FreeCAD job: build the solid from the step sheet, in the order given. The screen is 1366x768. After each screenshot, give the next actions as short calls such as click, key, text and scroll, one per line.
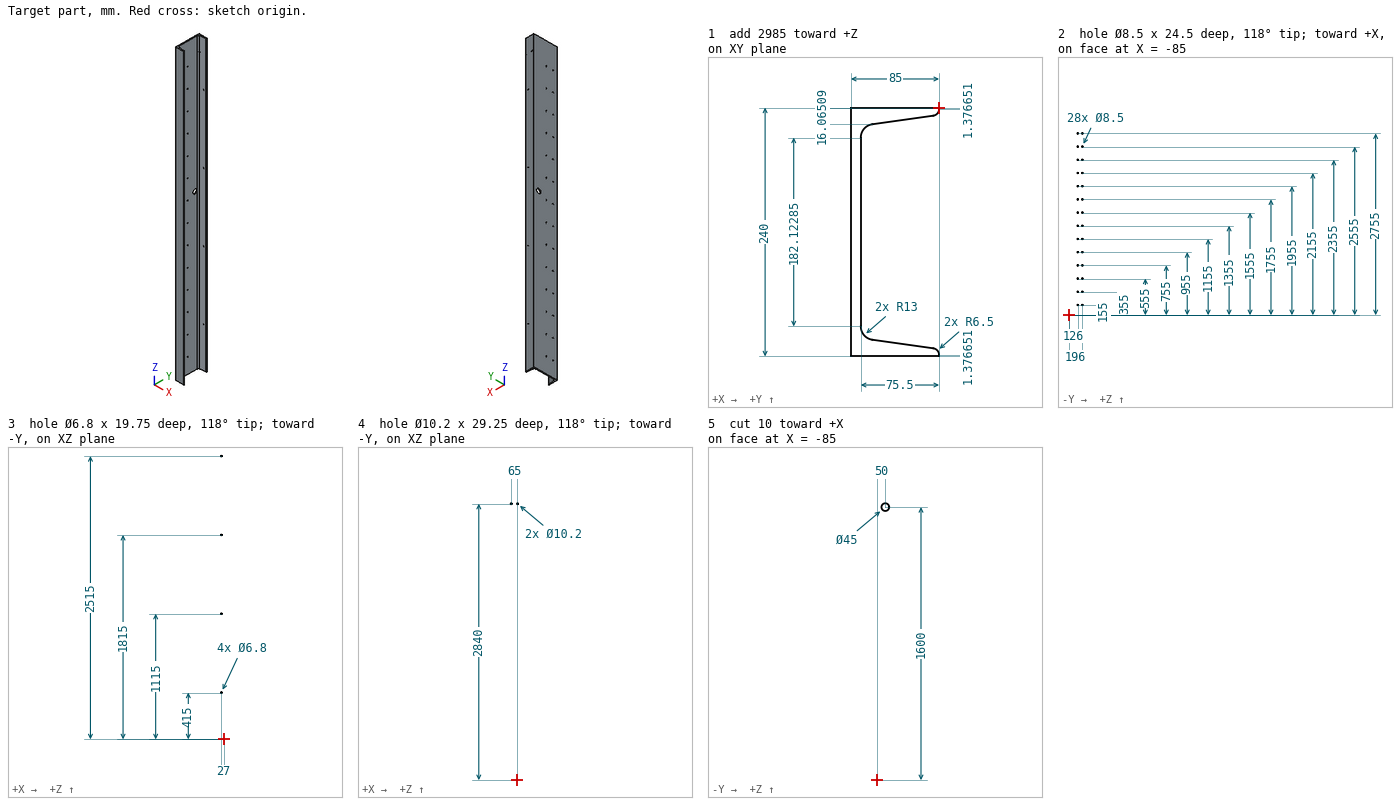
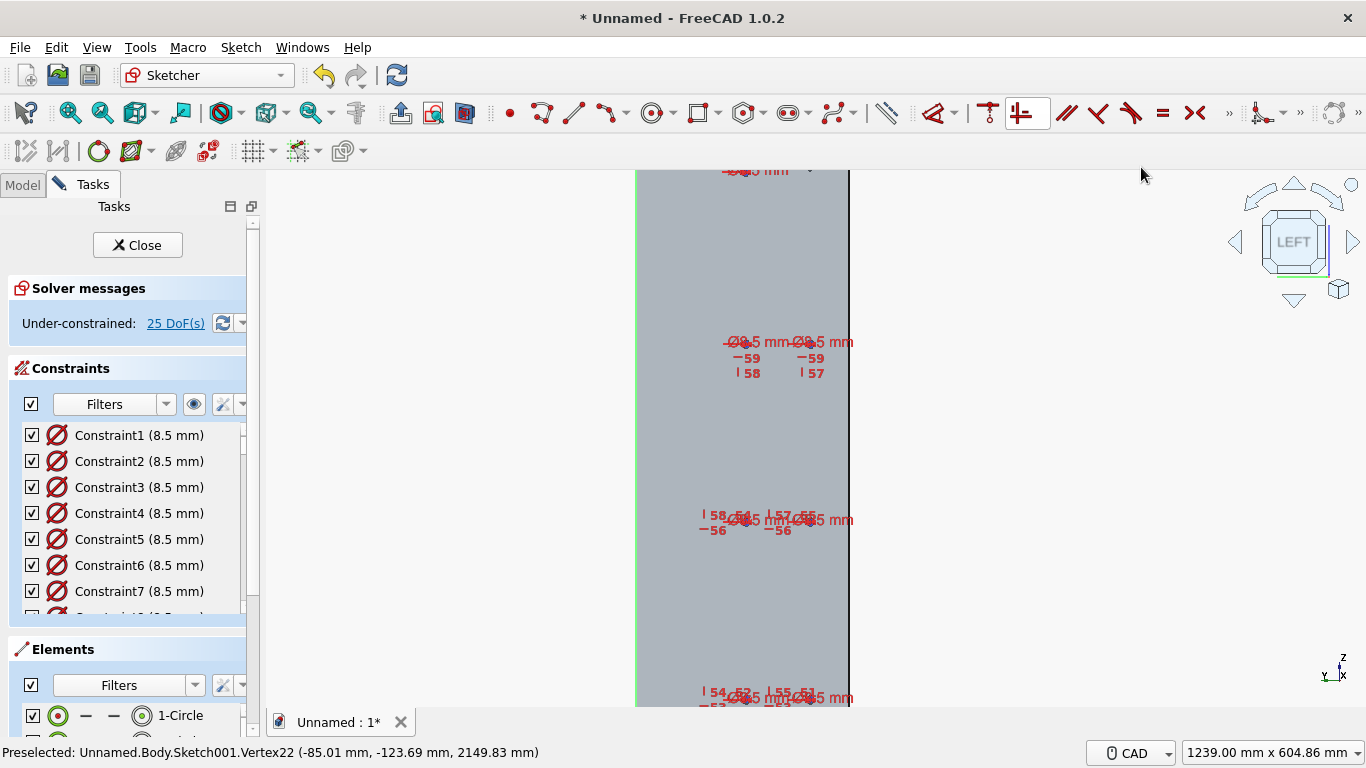
scroll(751, 346, down, 10)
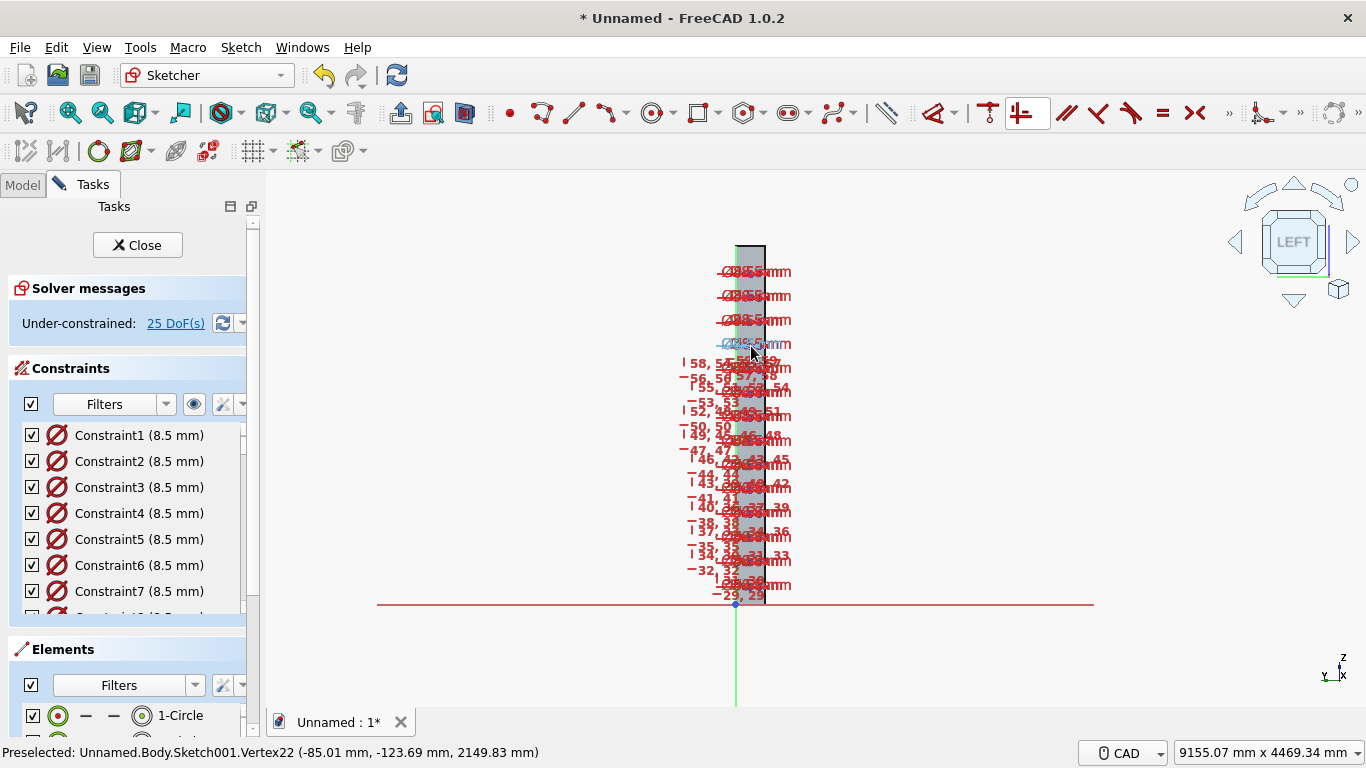
scroll(751, 346, up, 2)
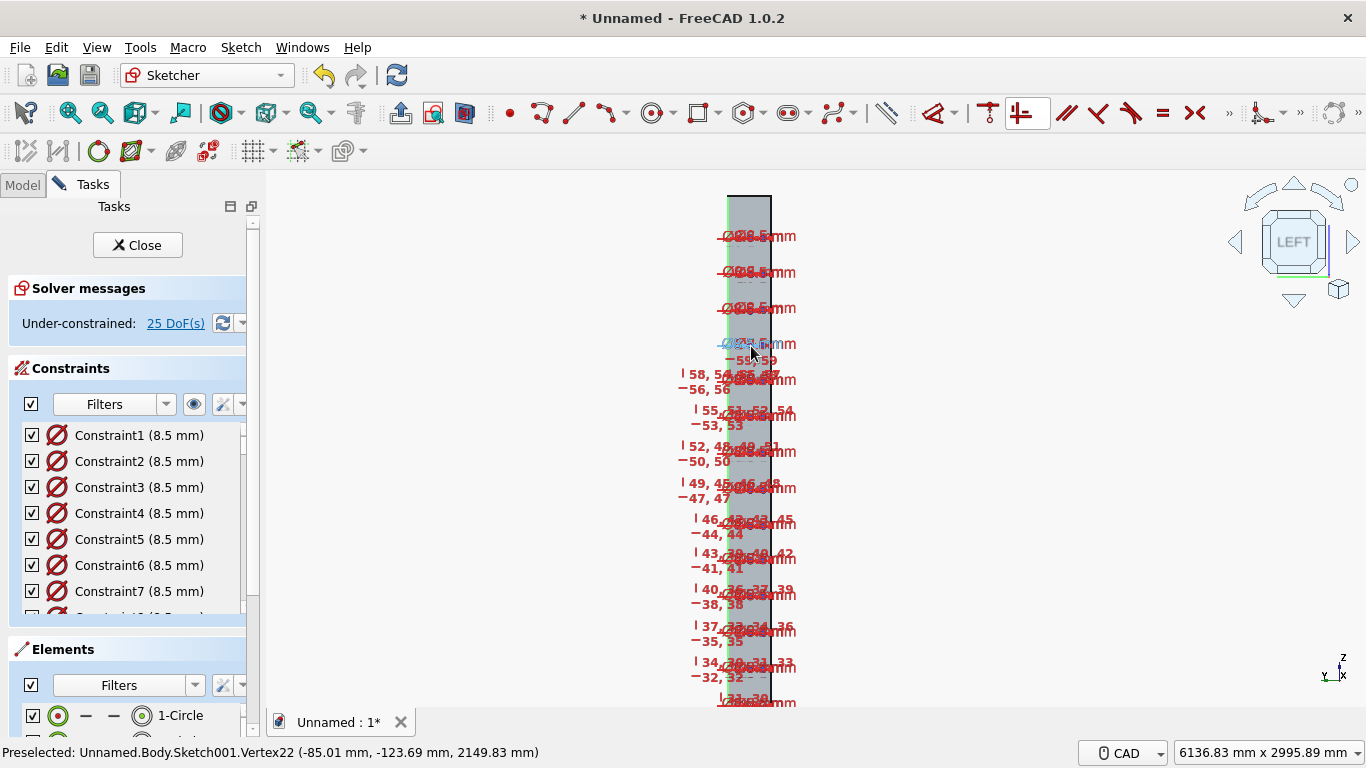
click(750, 346)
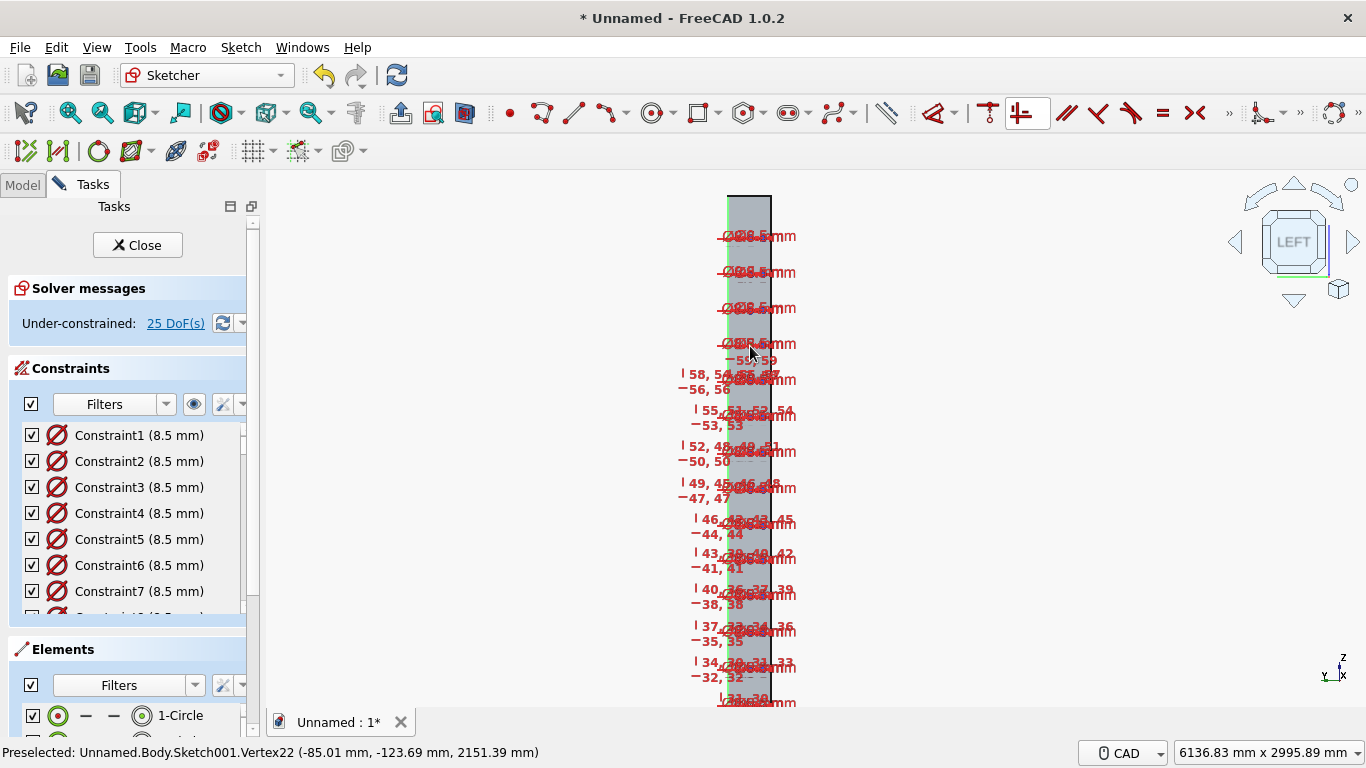
click(750, 311)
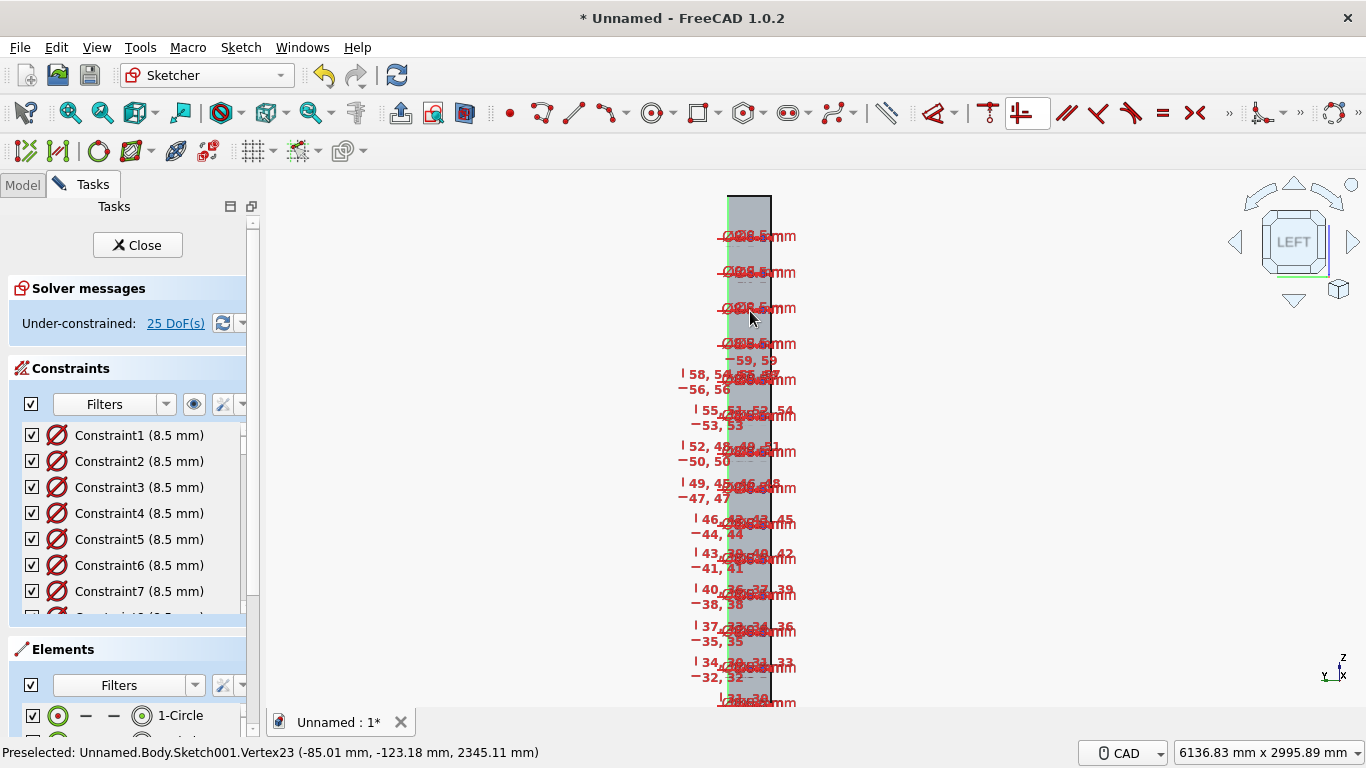
key(v)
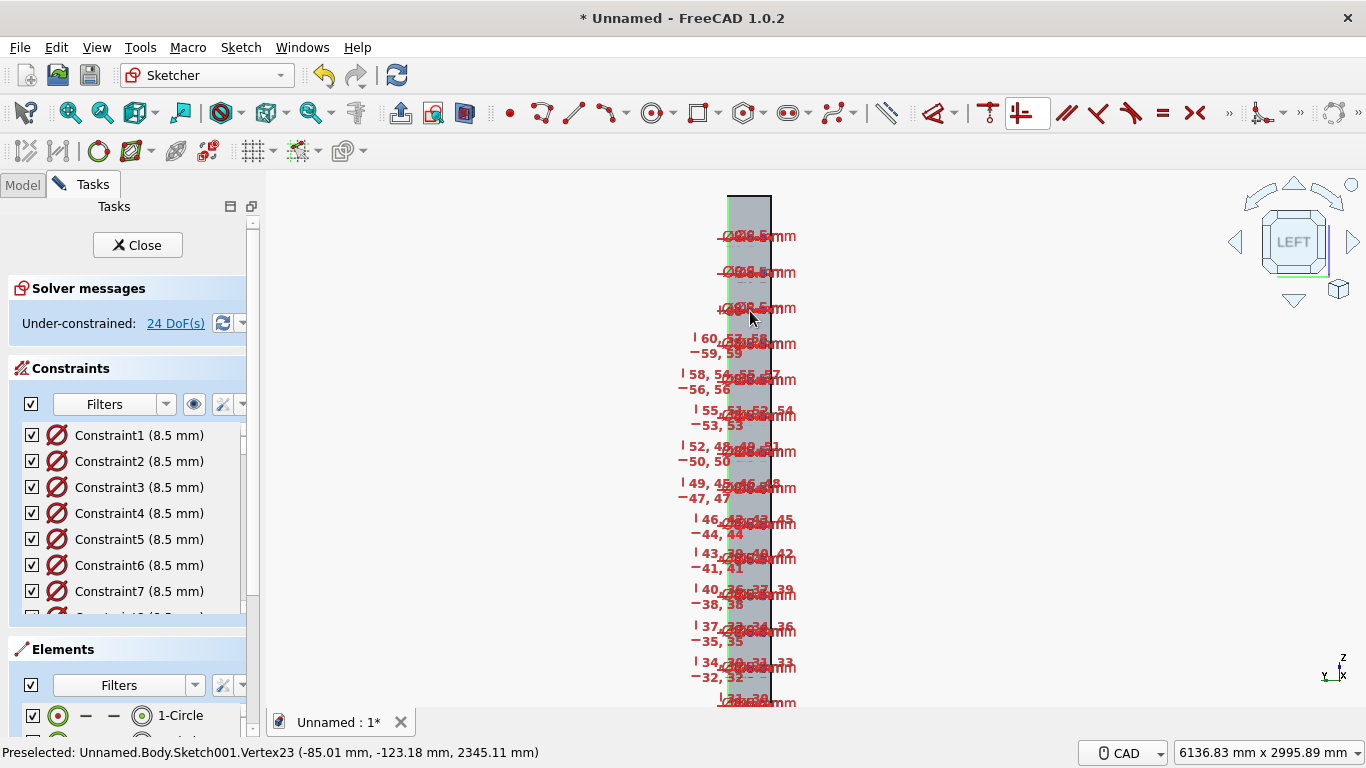
click(763, 346)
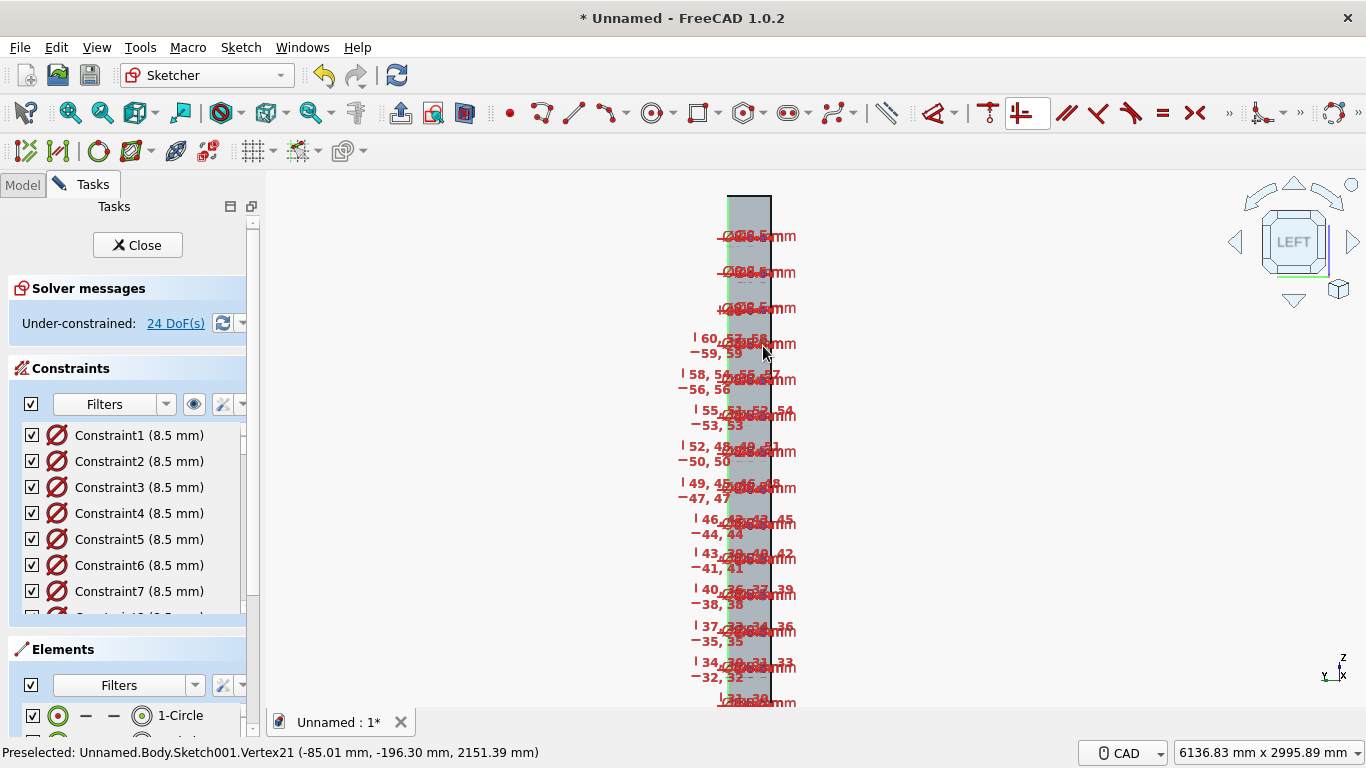
click(763, 310)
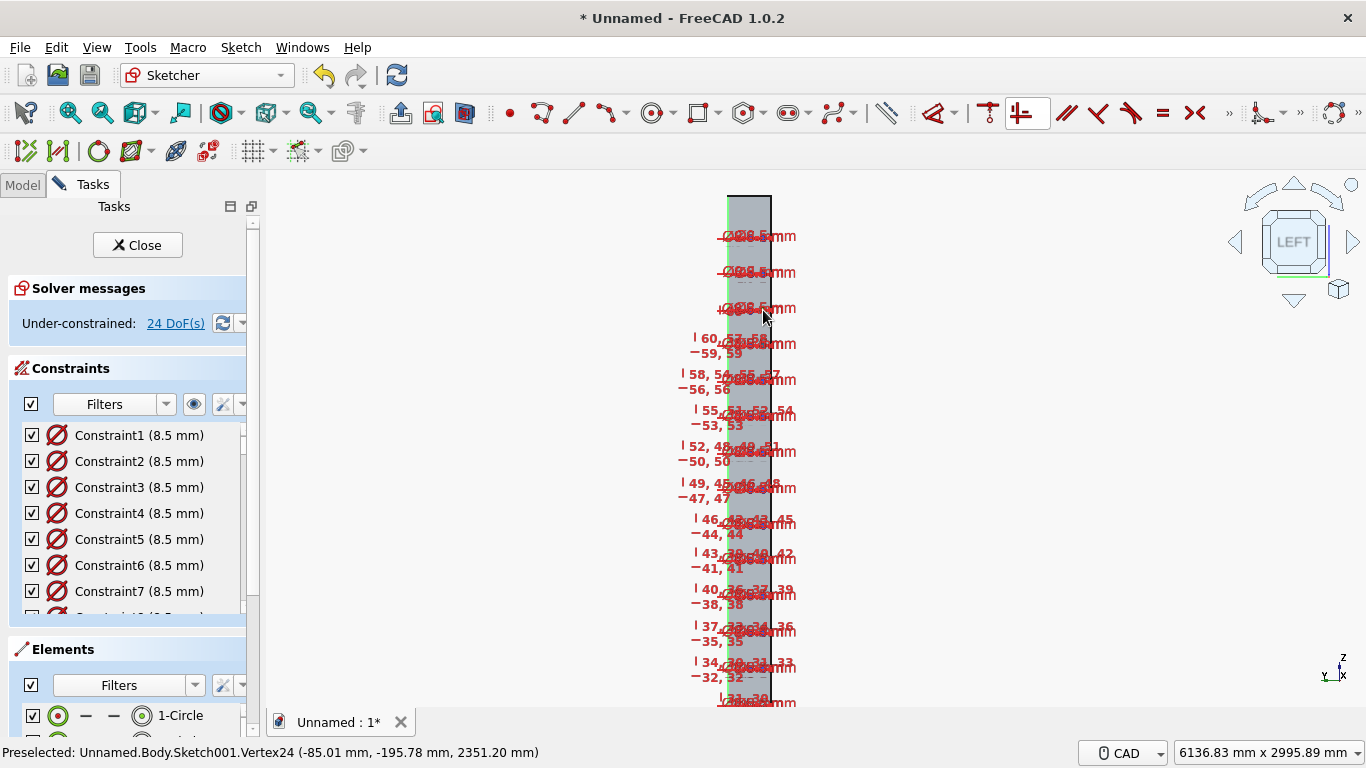
click(1044, 114)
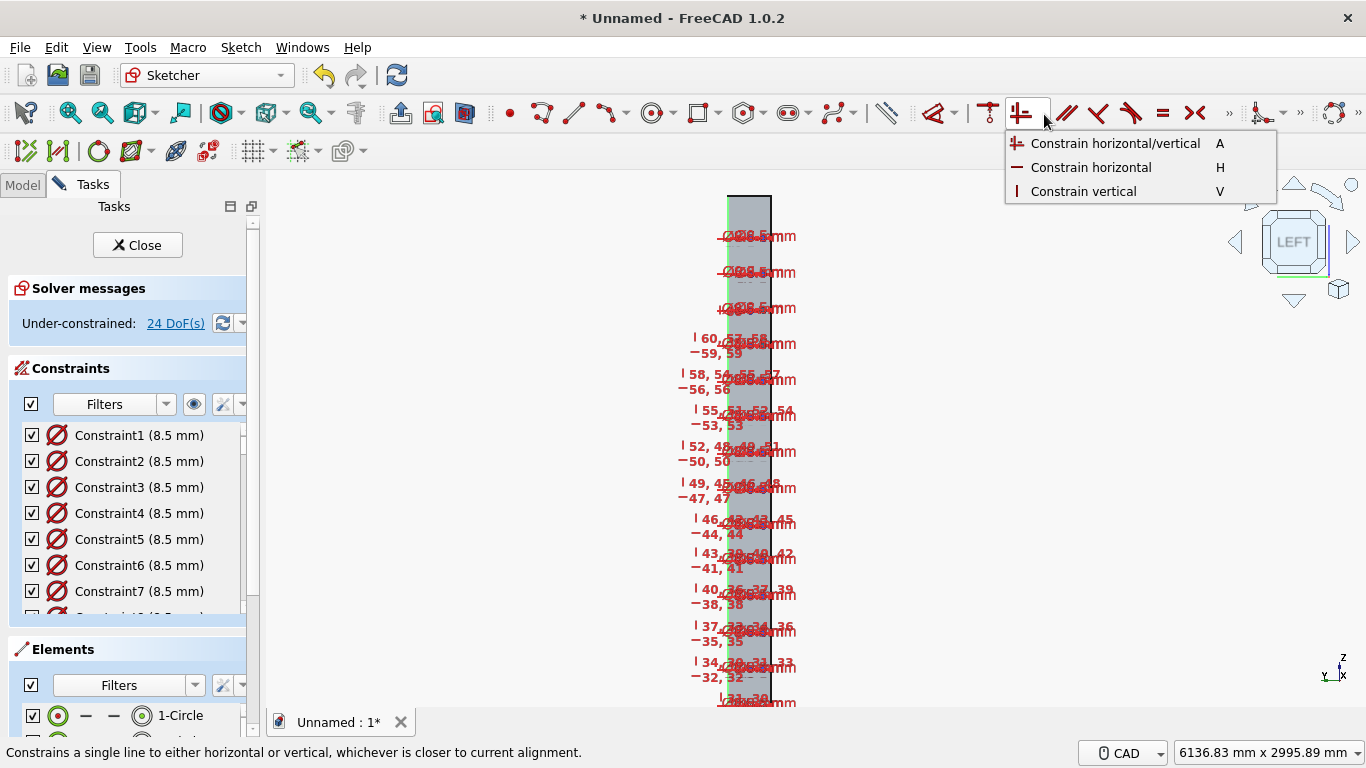
click(1141, 191)